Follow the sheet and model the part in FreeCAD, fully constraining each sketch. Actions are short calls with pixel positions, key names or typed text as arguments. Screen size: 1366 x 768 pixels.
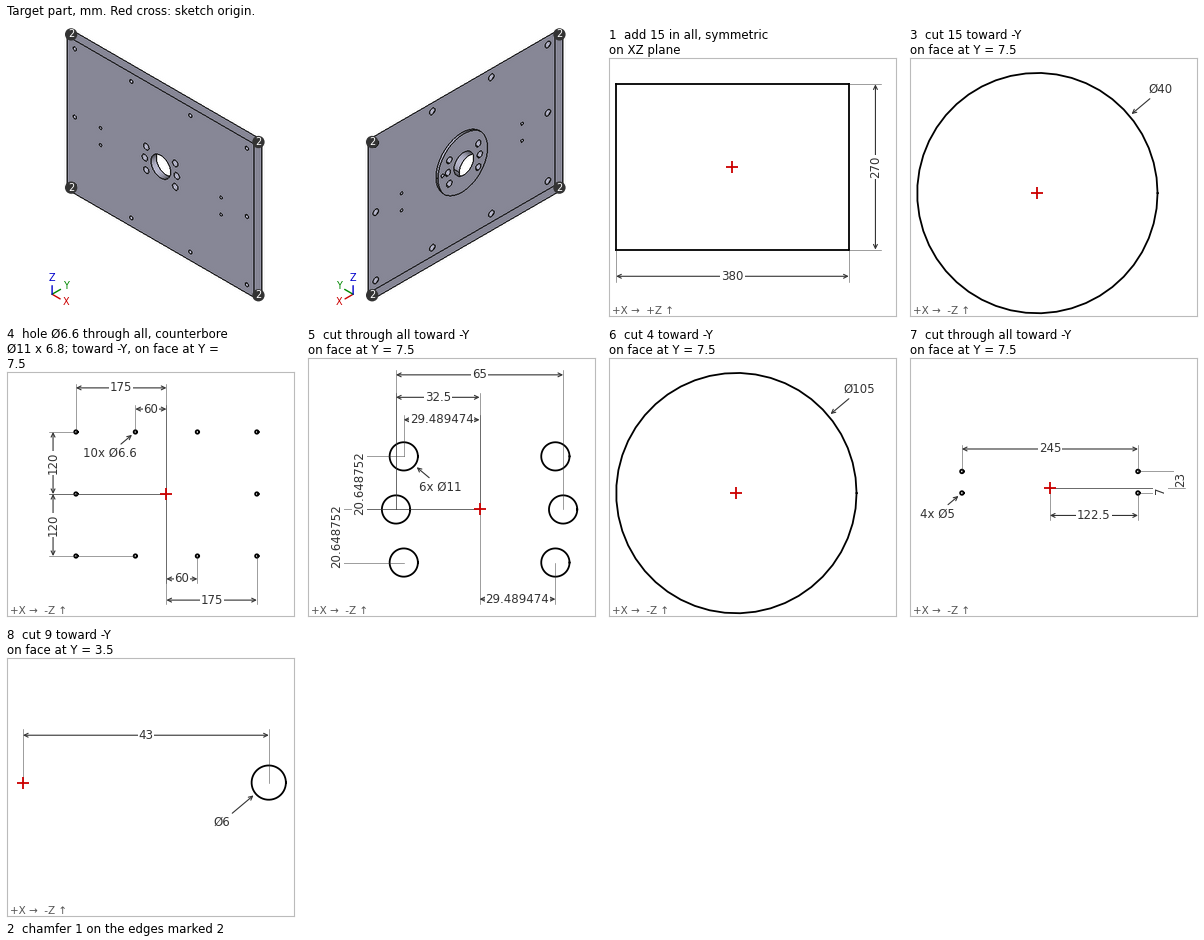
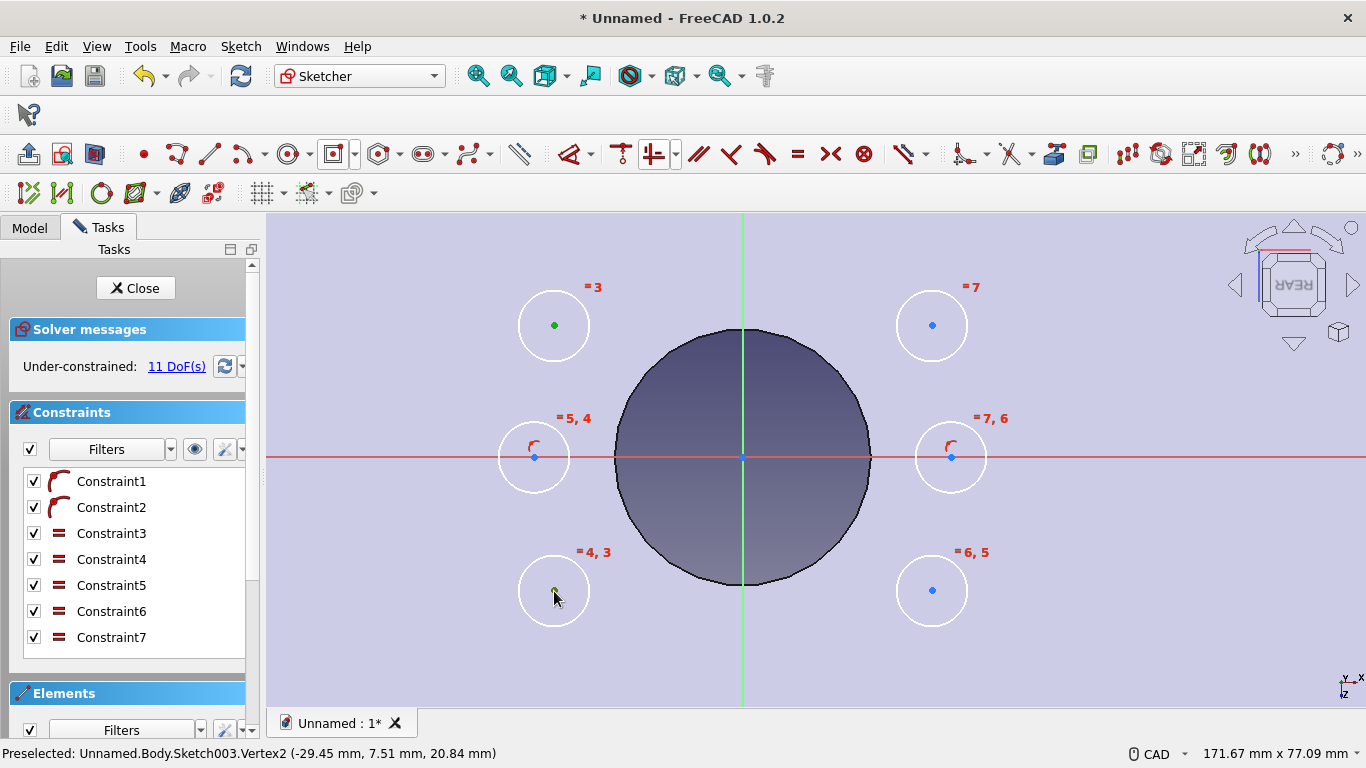
key(v)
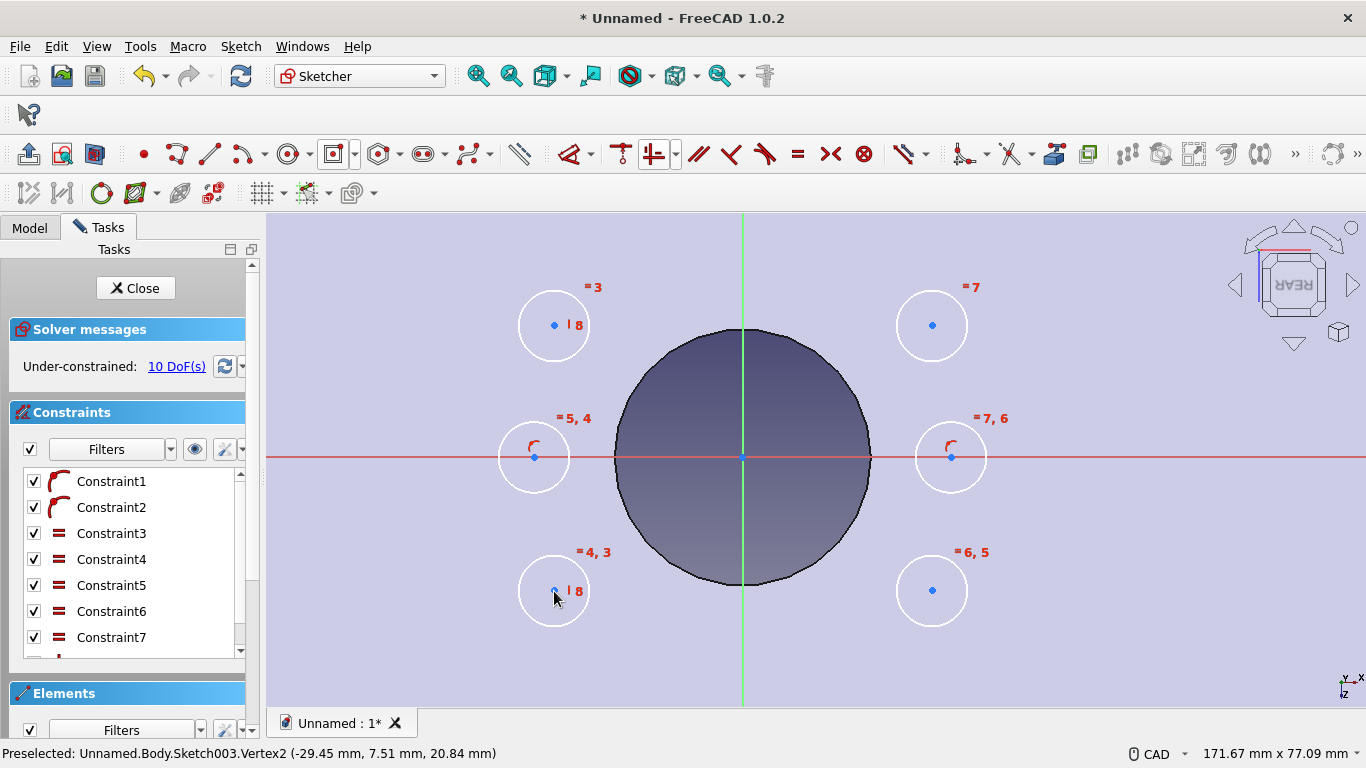
click(554, 591)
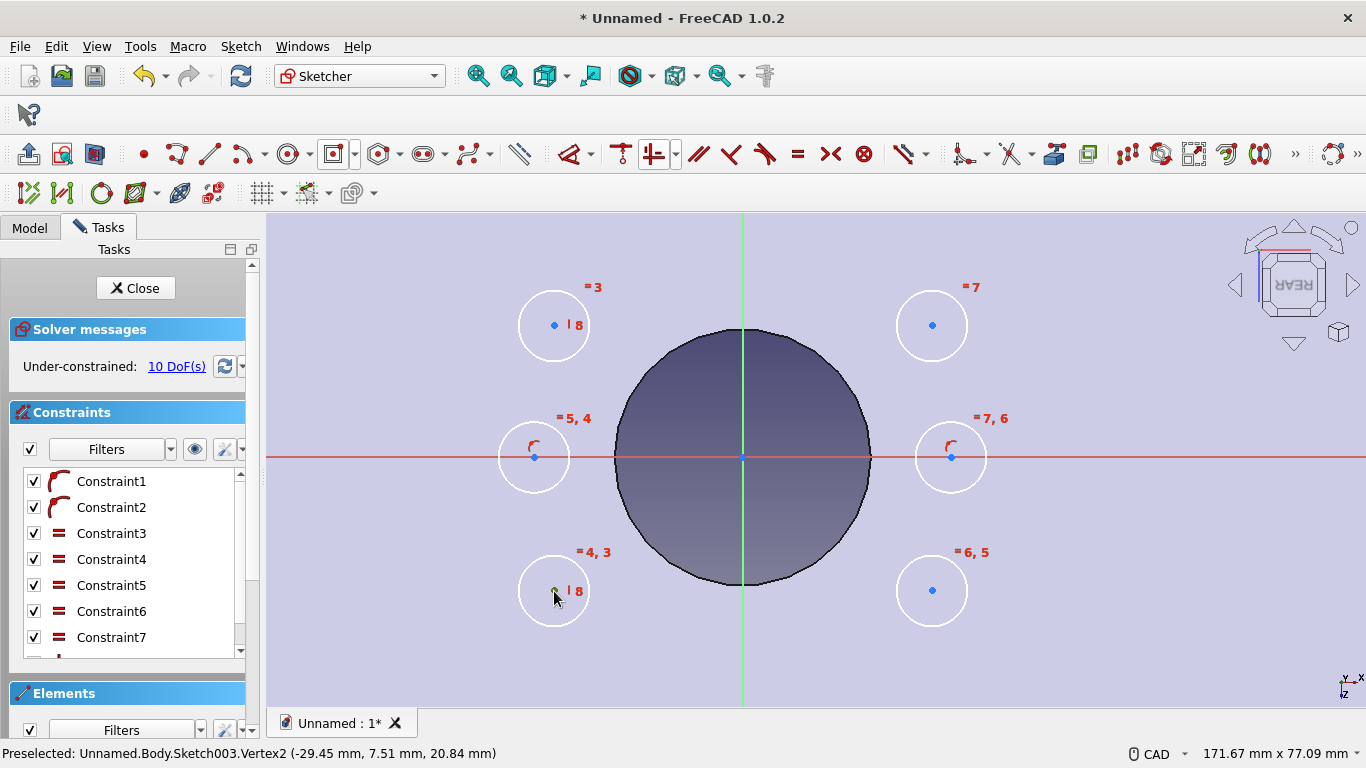
click(932, 591)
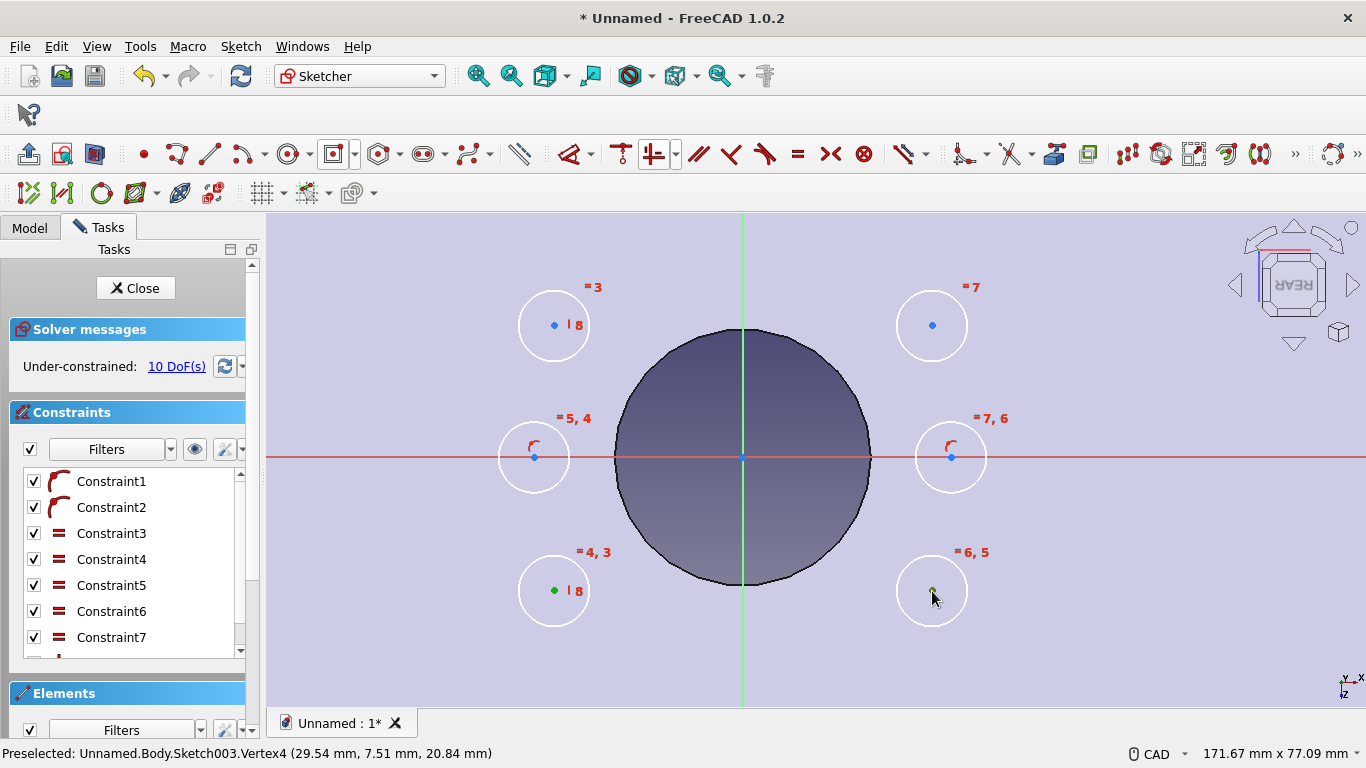
key(h)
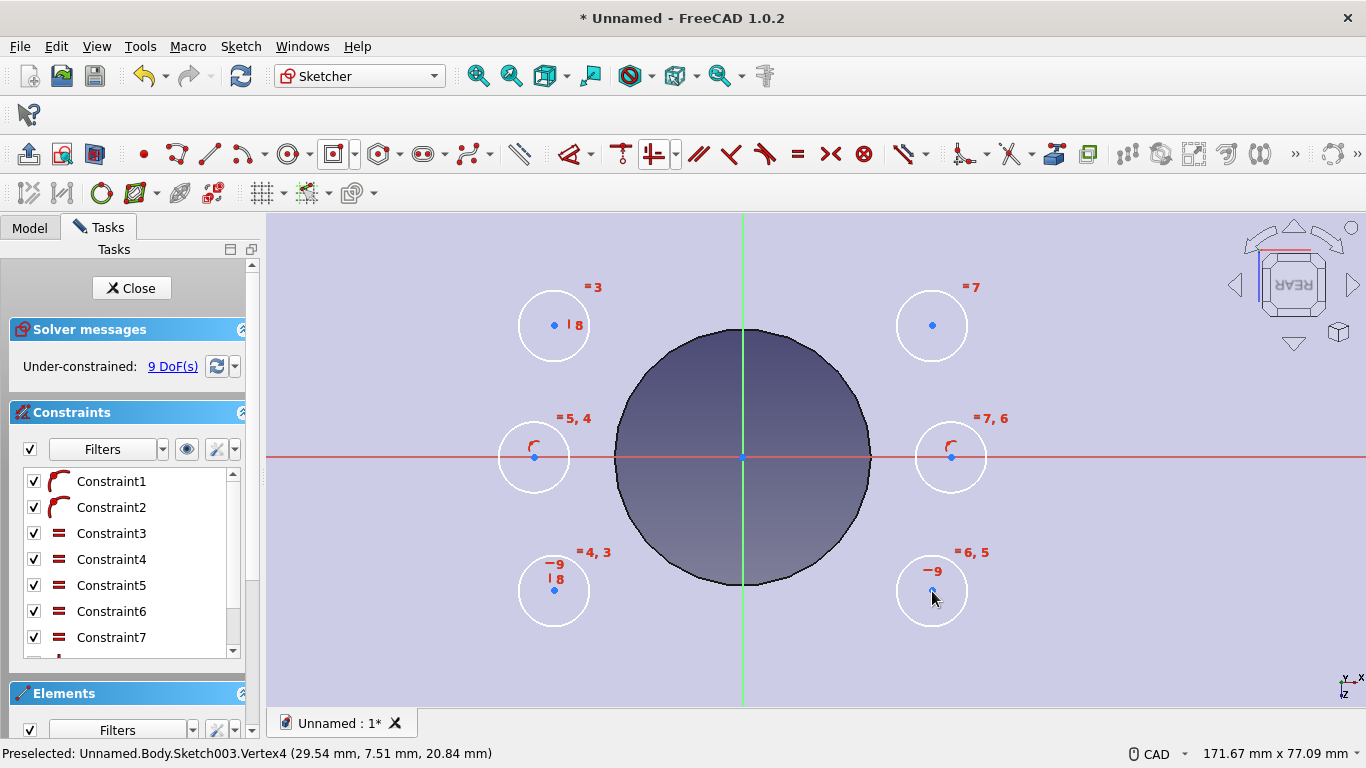
click(932, 591)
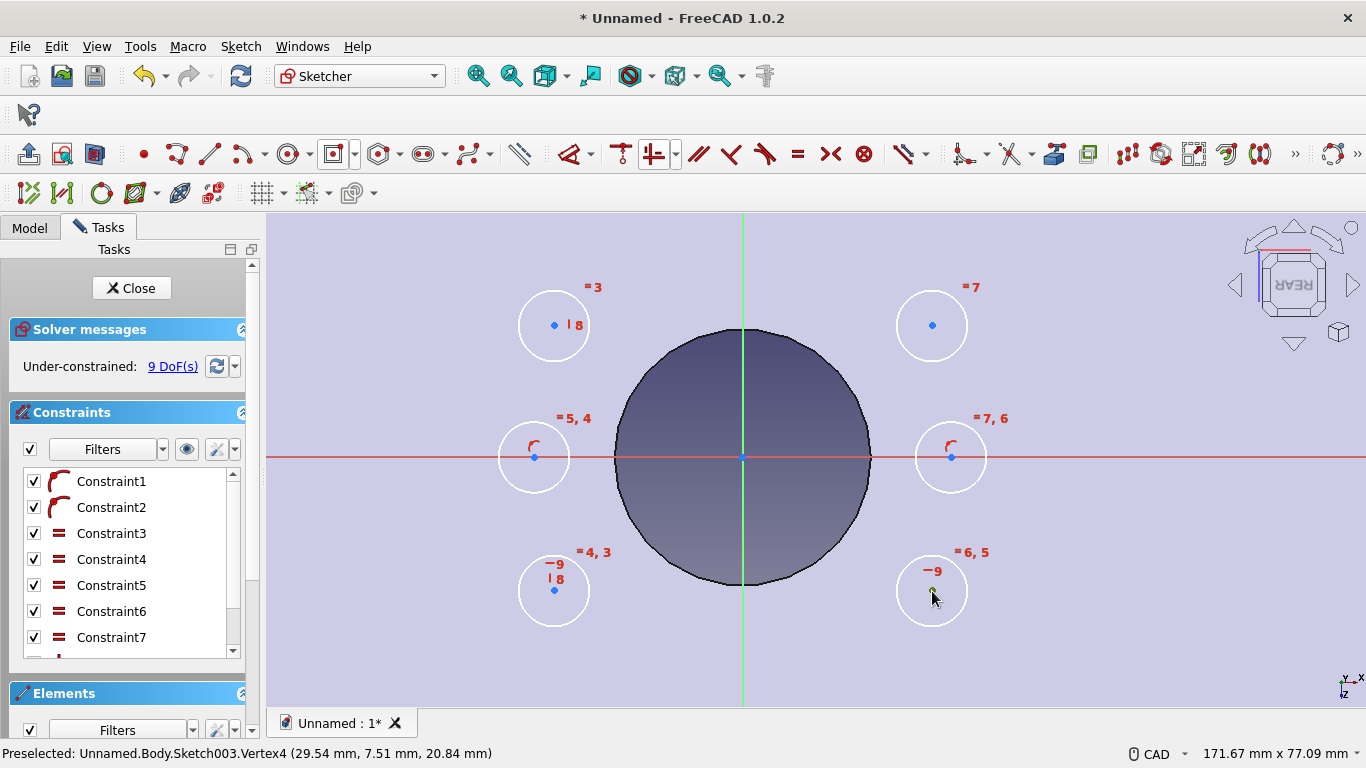
click(932, 326)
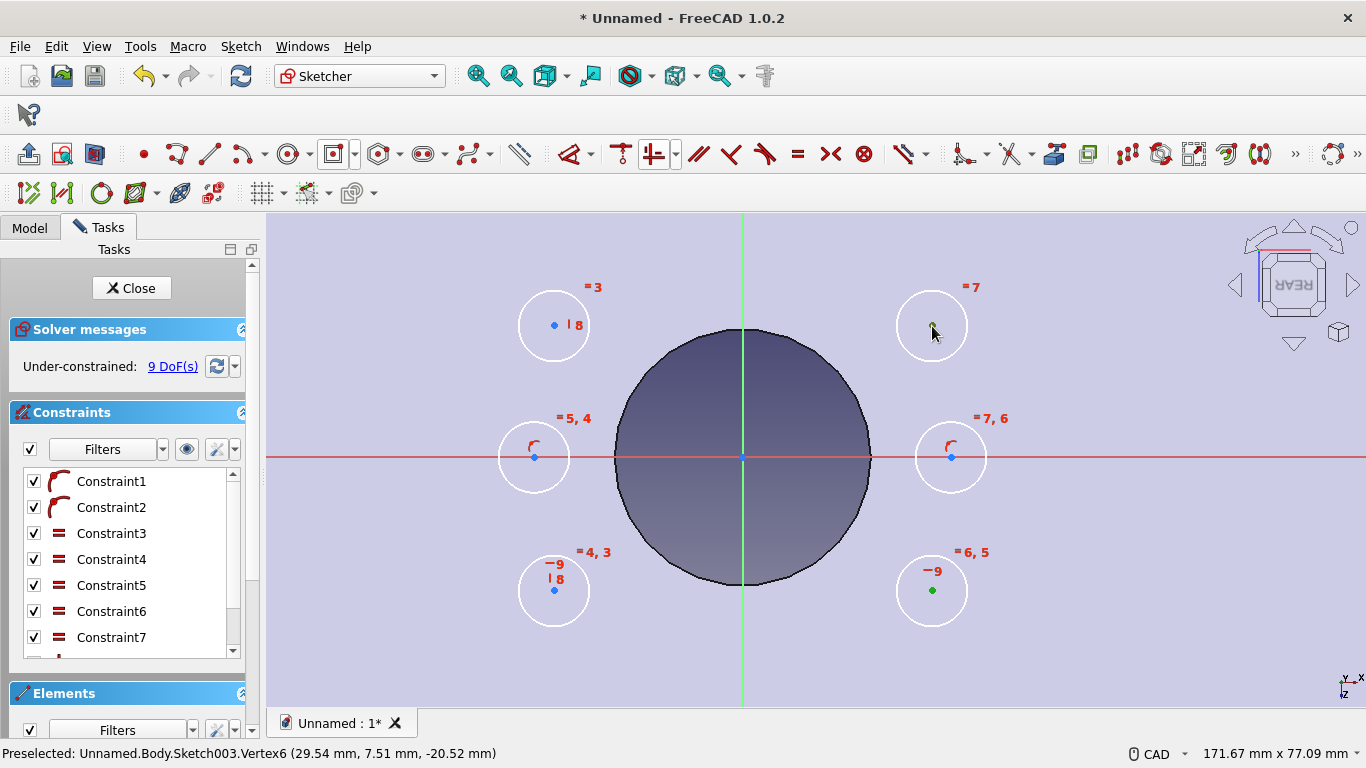
click(676, 154)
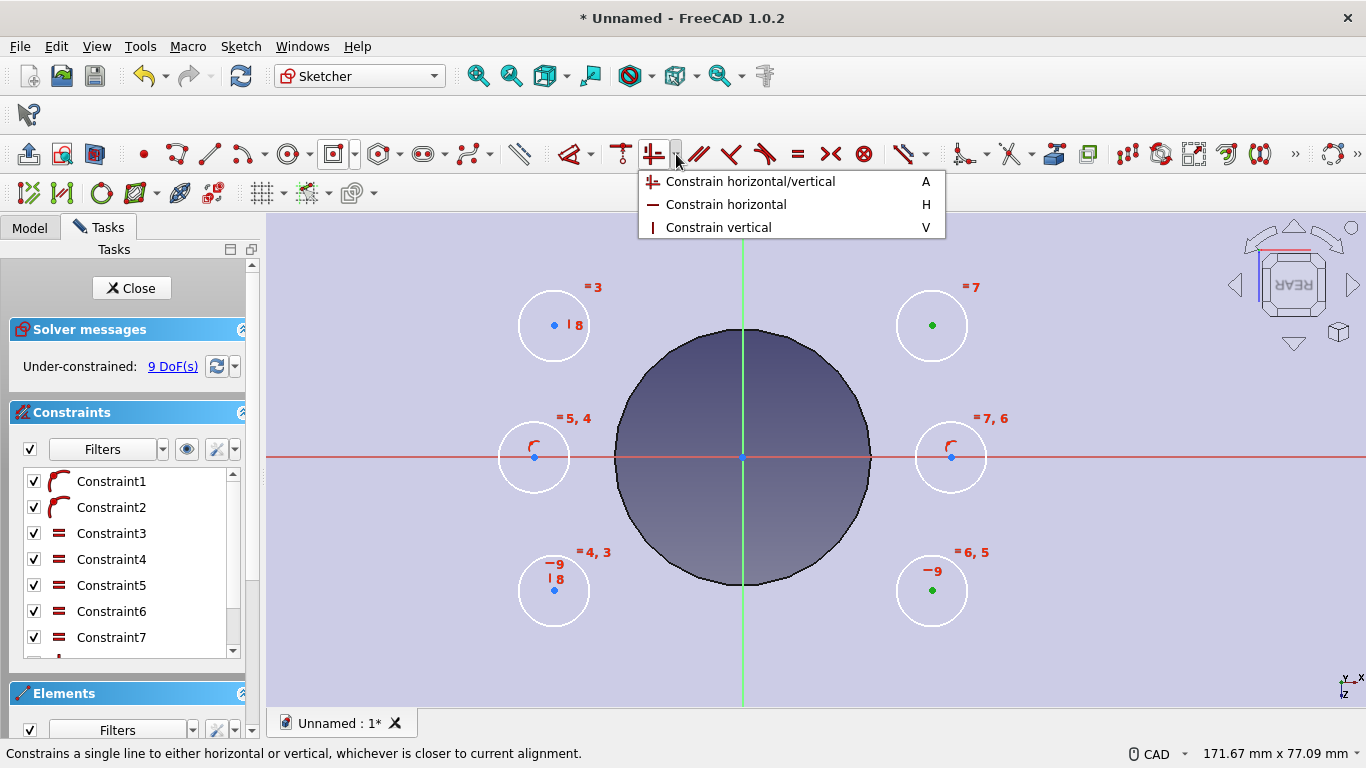
click(792, 228)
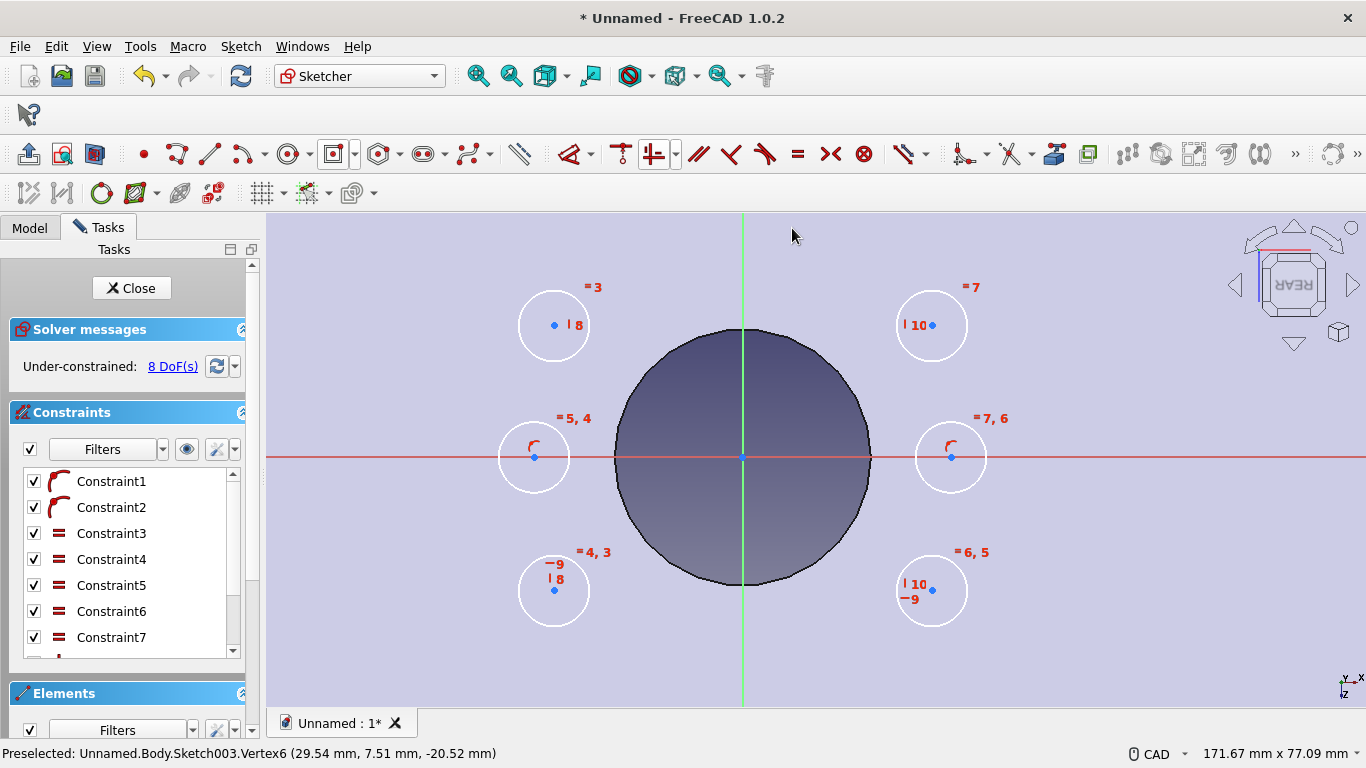
click(554, 326)